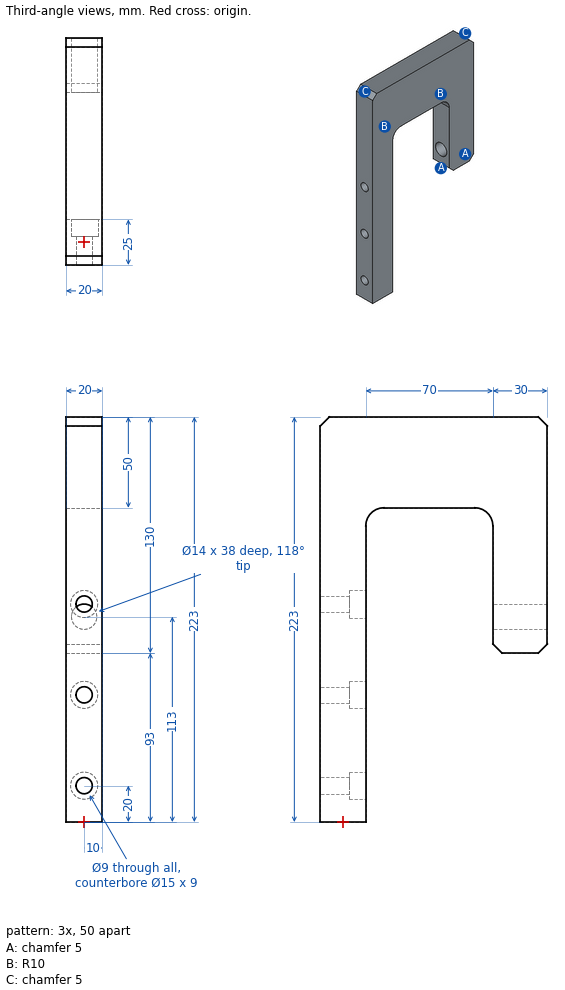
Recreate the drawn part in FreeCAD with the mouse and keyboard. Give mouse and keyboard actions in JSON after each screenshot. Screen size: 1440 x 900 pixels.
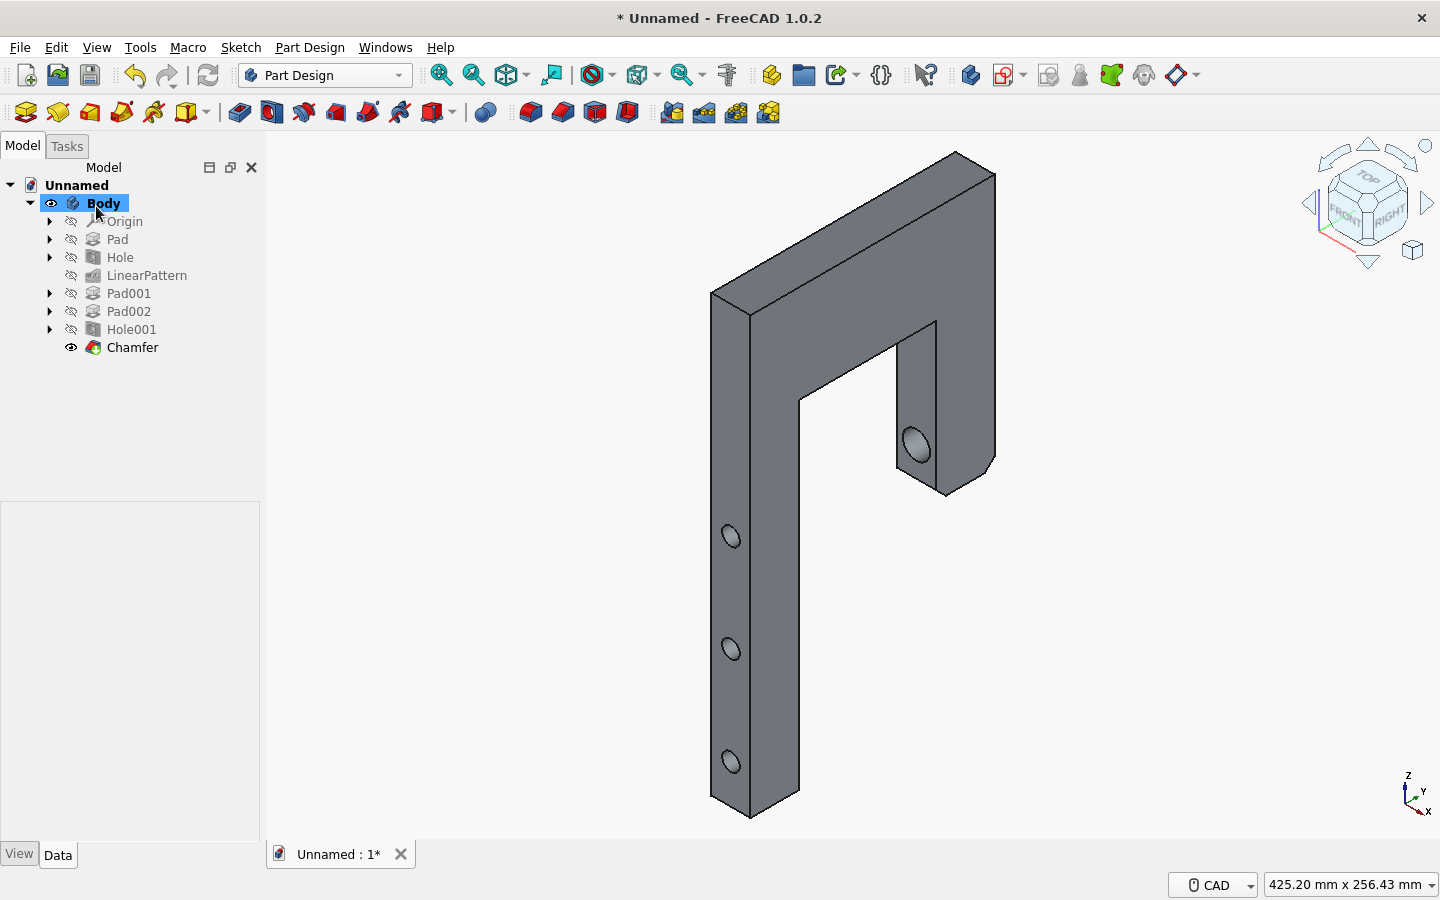
{"action": "key", "text": "2"}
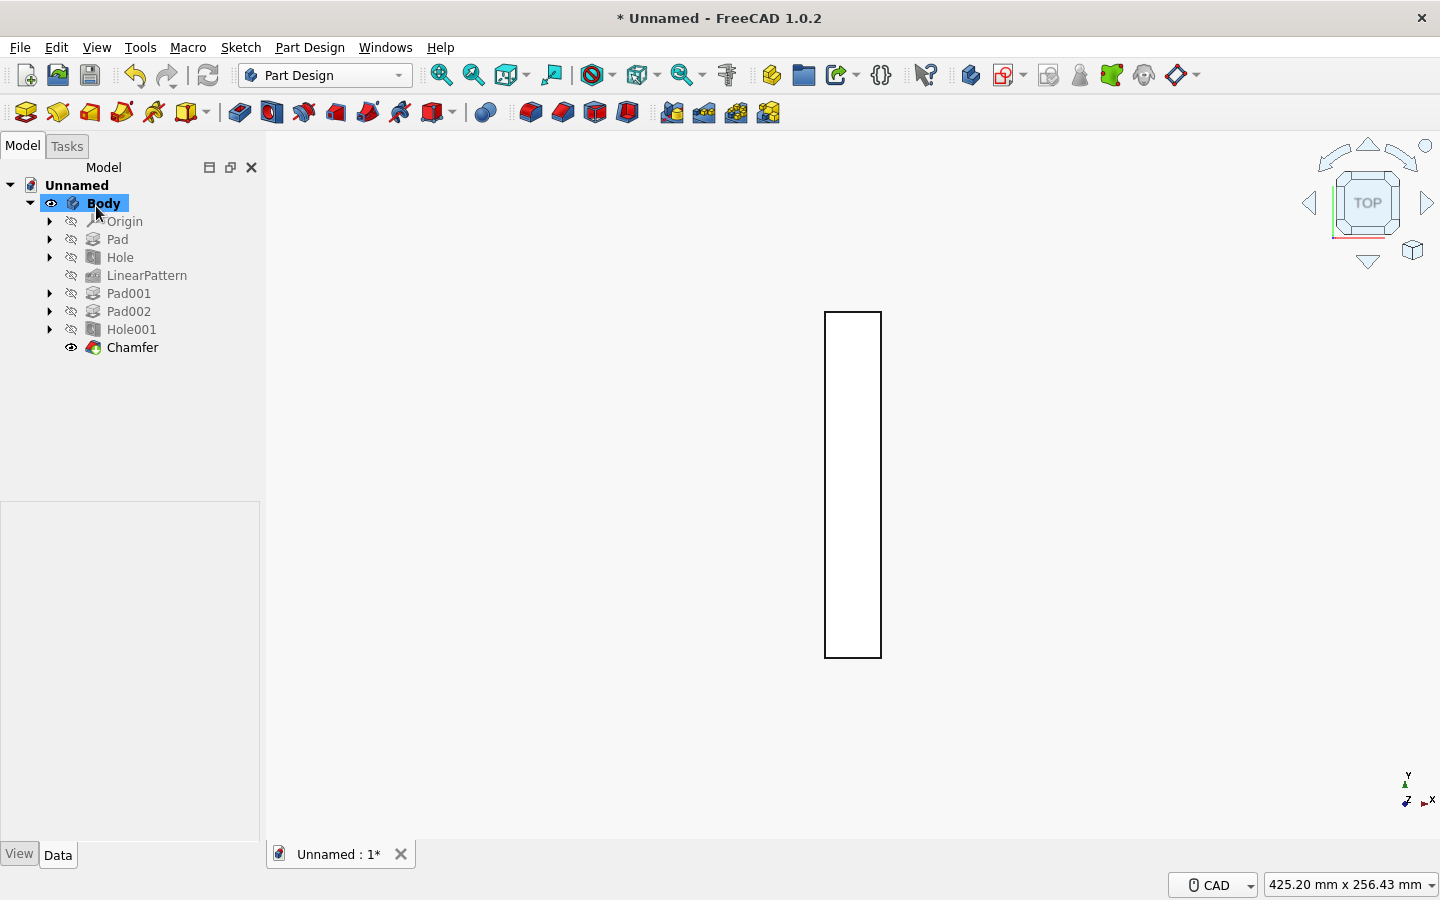
{"action": "key", "text": "1"}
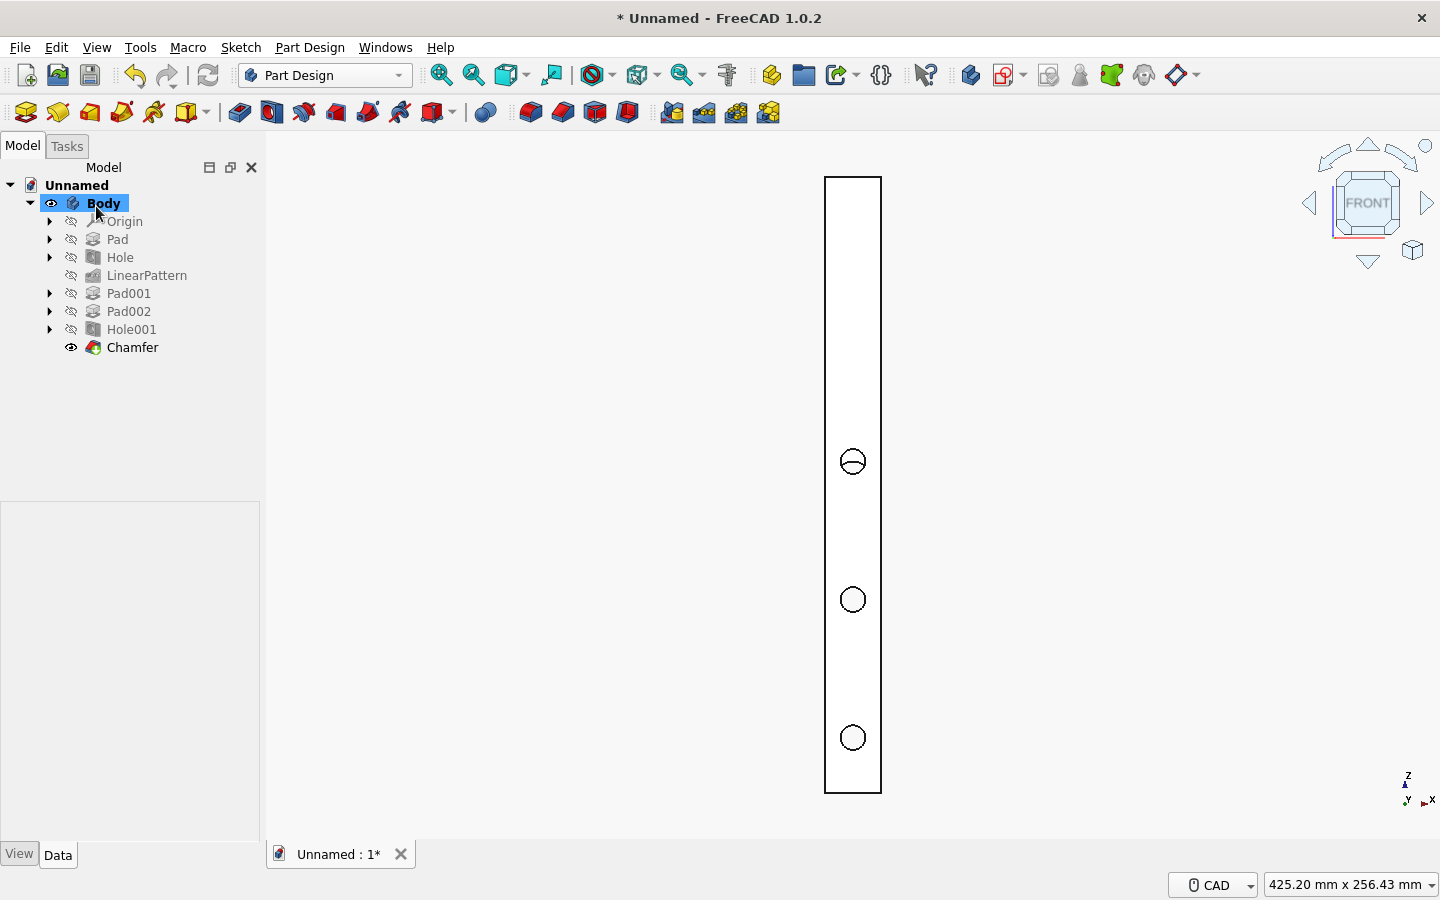
{"action": "key", "text": "3"}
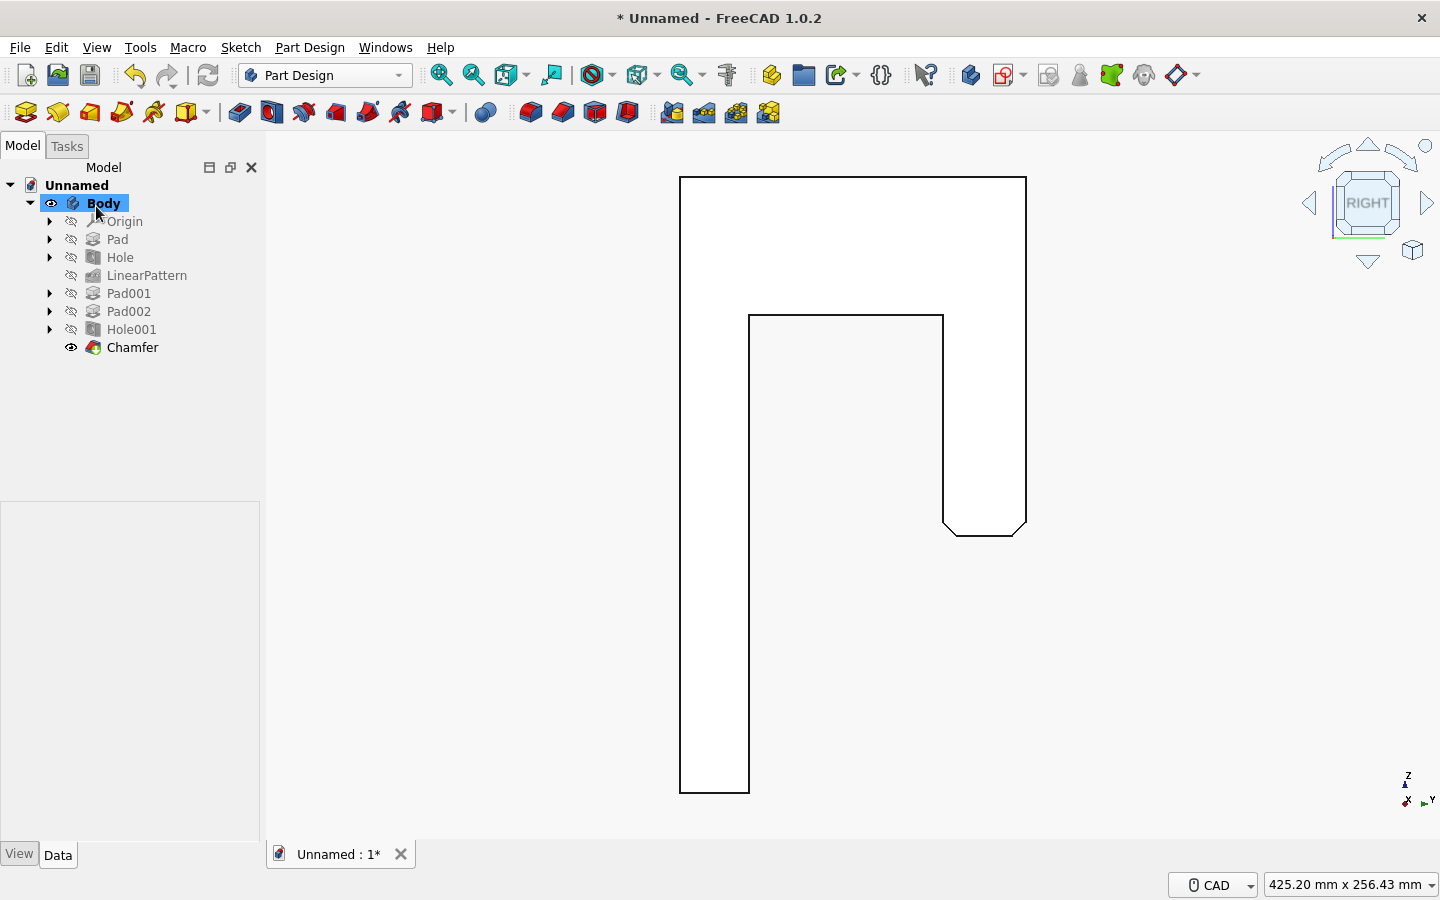
{"action": "key", "text": "5"}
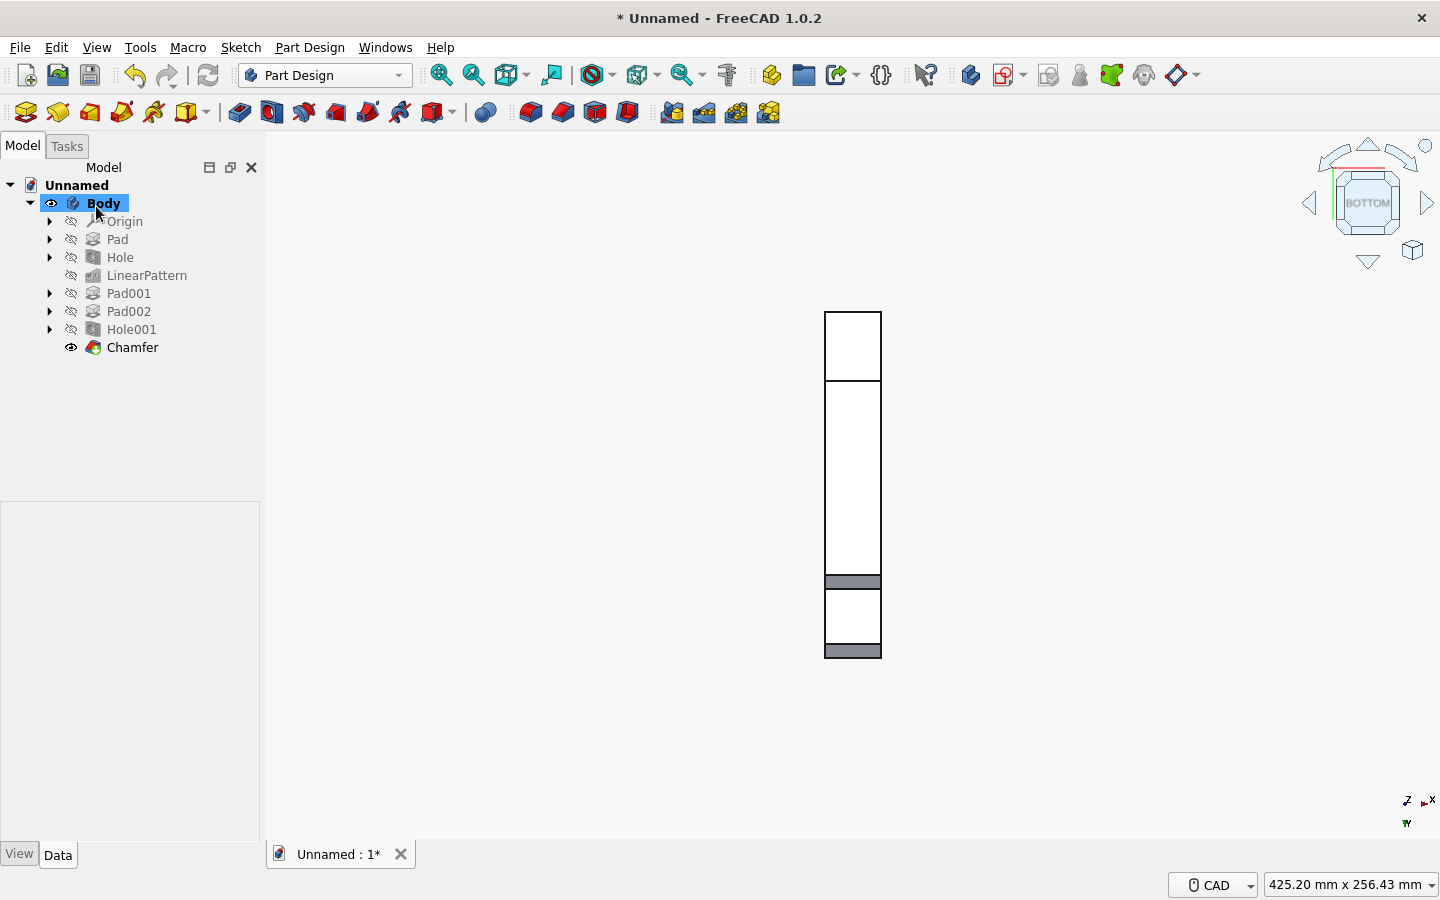
{"action": "key", "text": "4"}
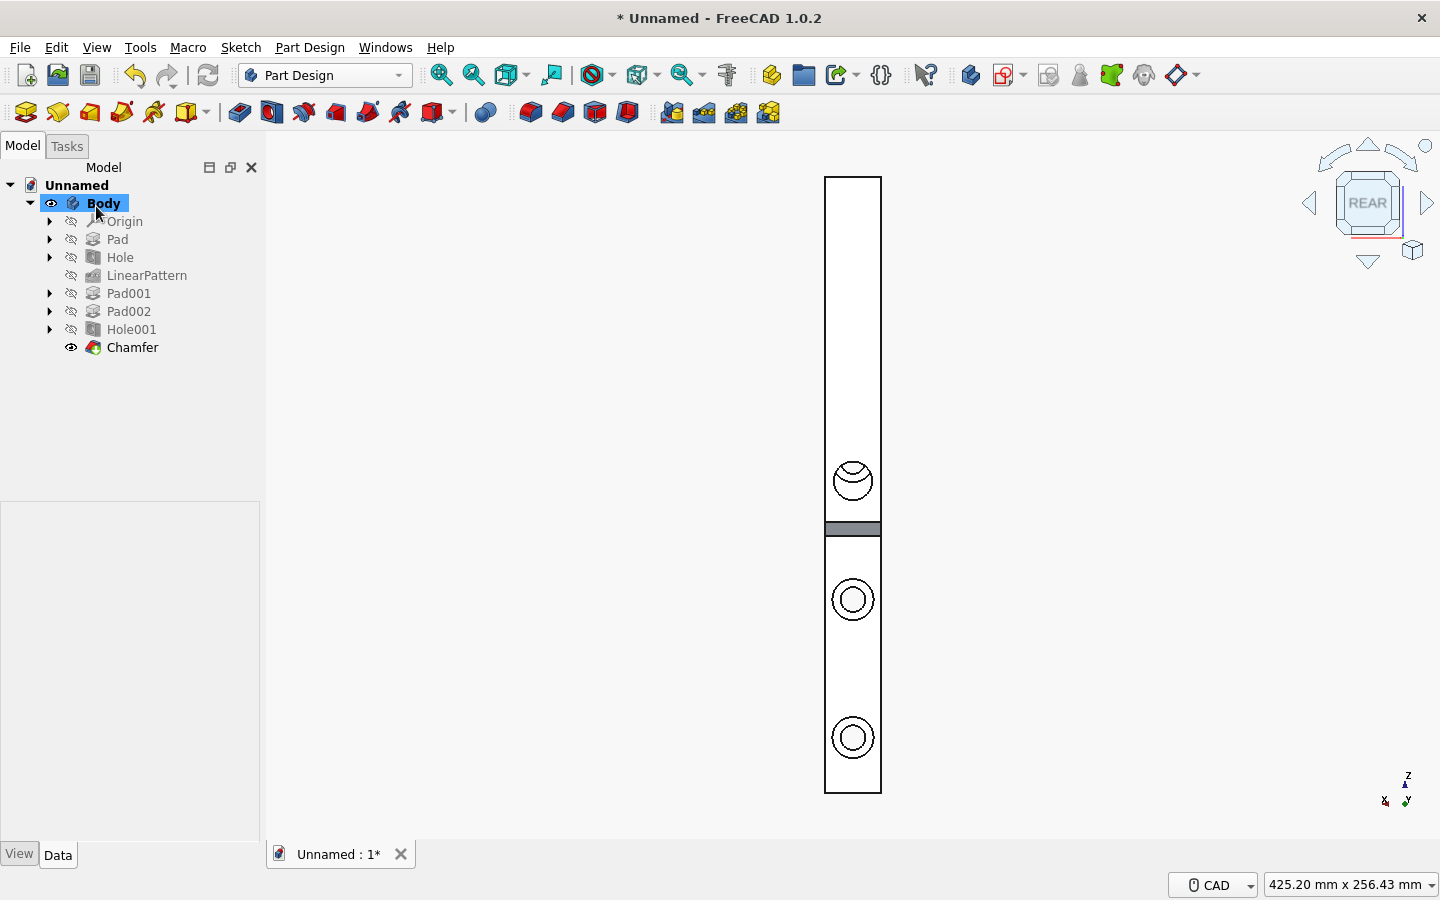
{"action": "key", "text": "6"}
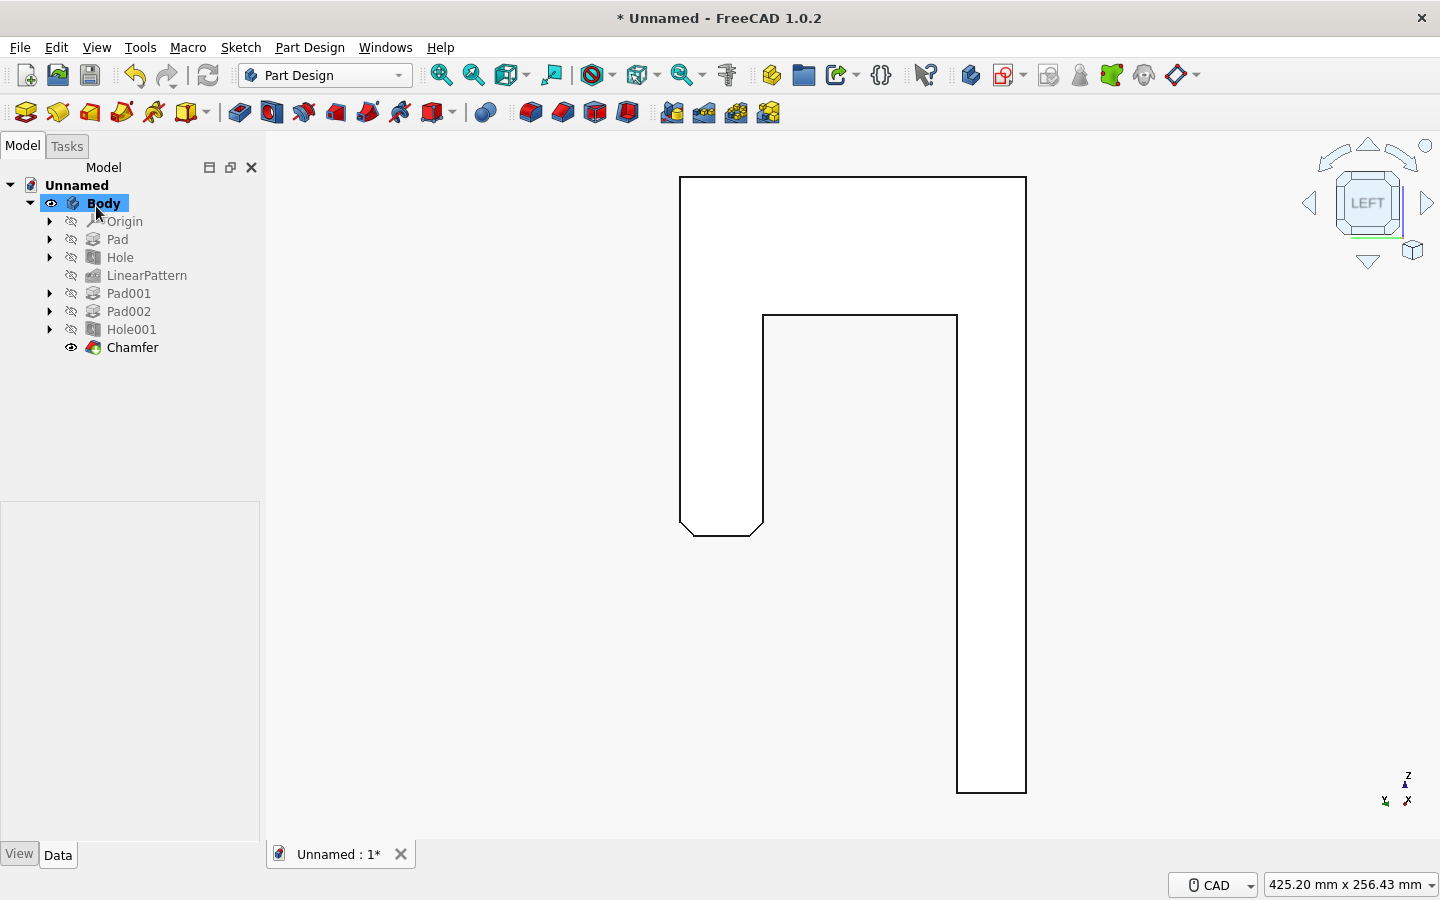
{"action": "key", "text": "v 3"}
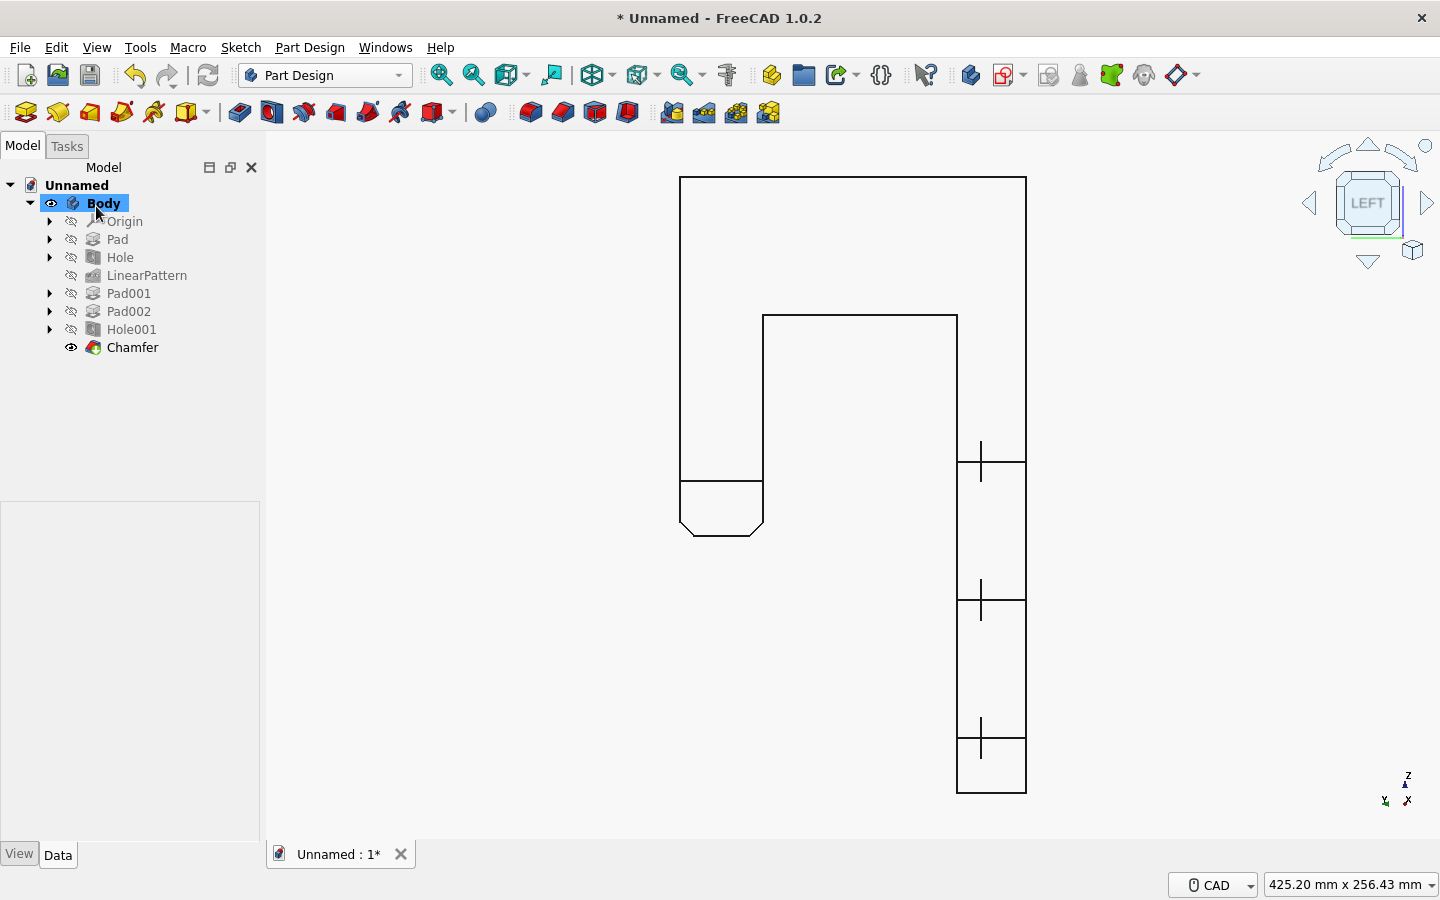
{"action": "key", "text": "0"}